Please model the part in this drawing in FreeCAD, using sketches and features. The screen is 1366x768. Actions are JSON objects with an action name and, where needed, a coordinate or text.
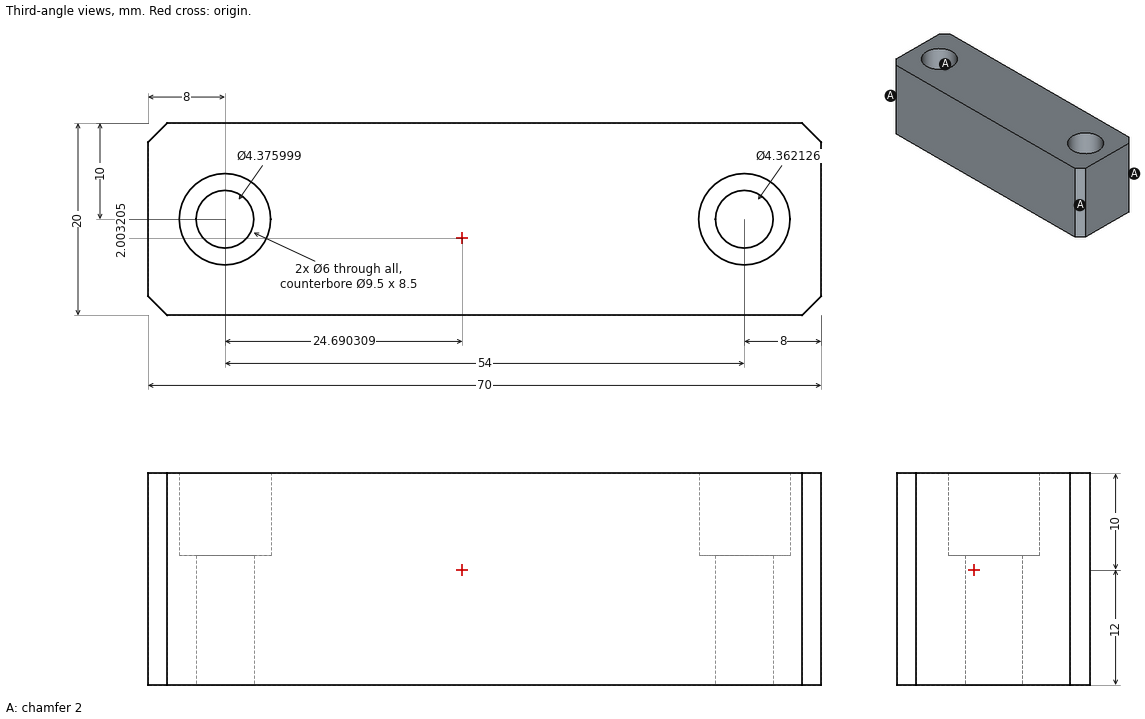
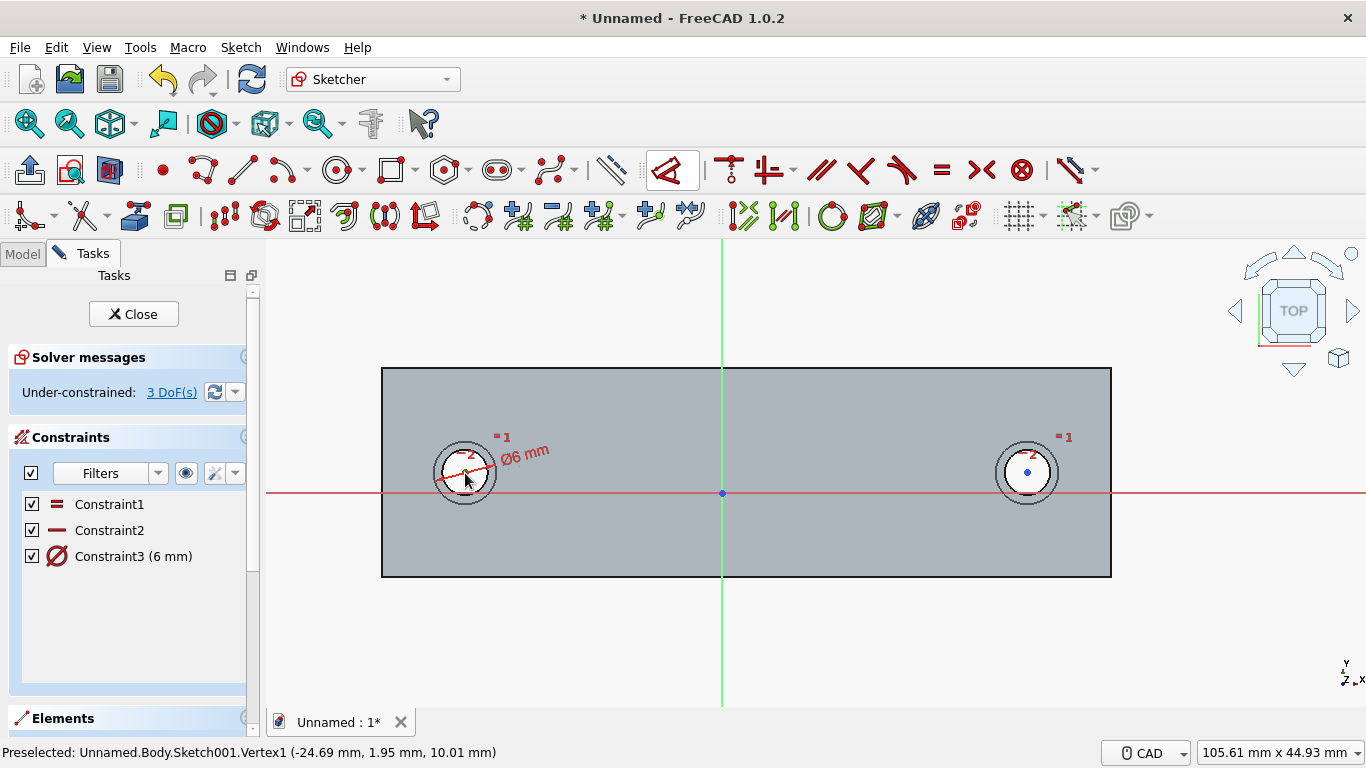
{"action": "left_click", "coordinate": [1027, 473]}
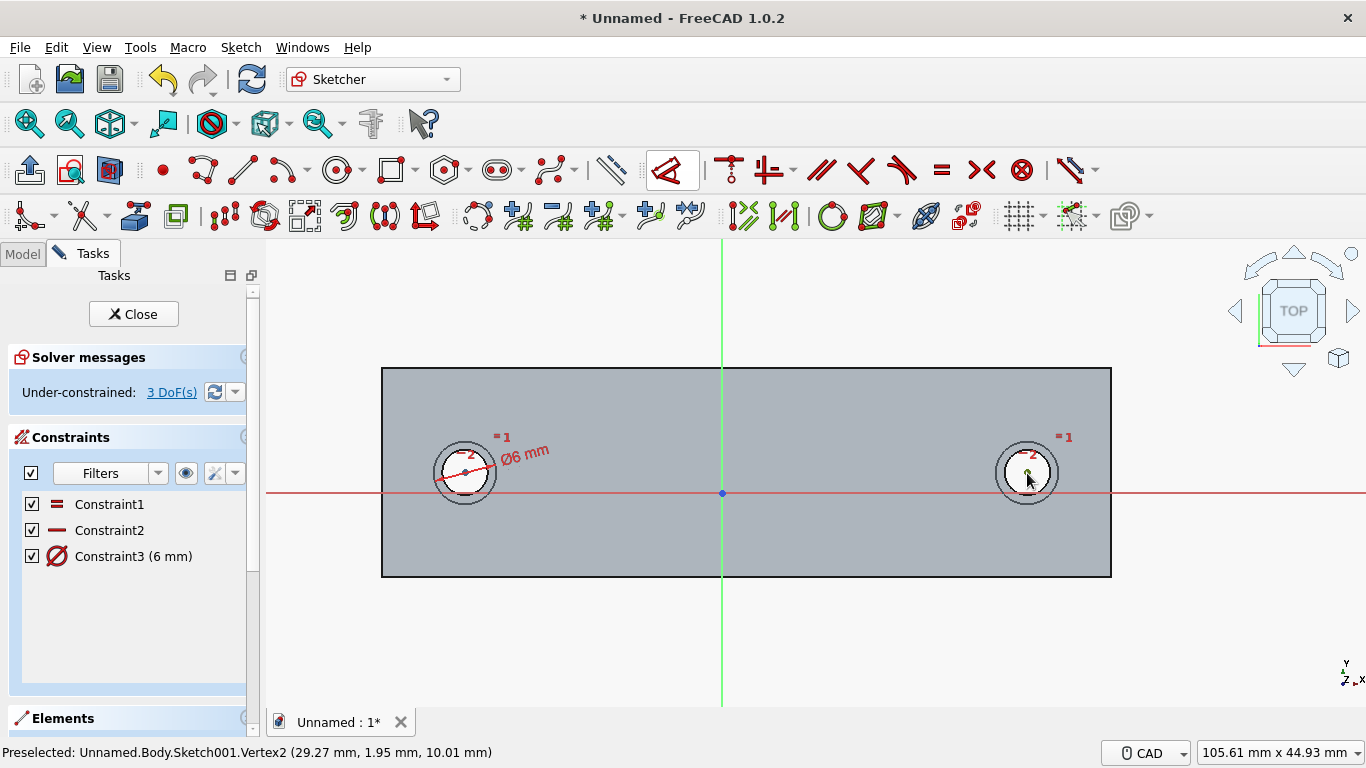
{"action": "key", "text": "l"}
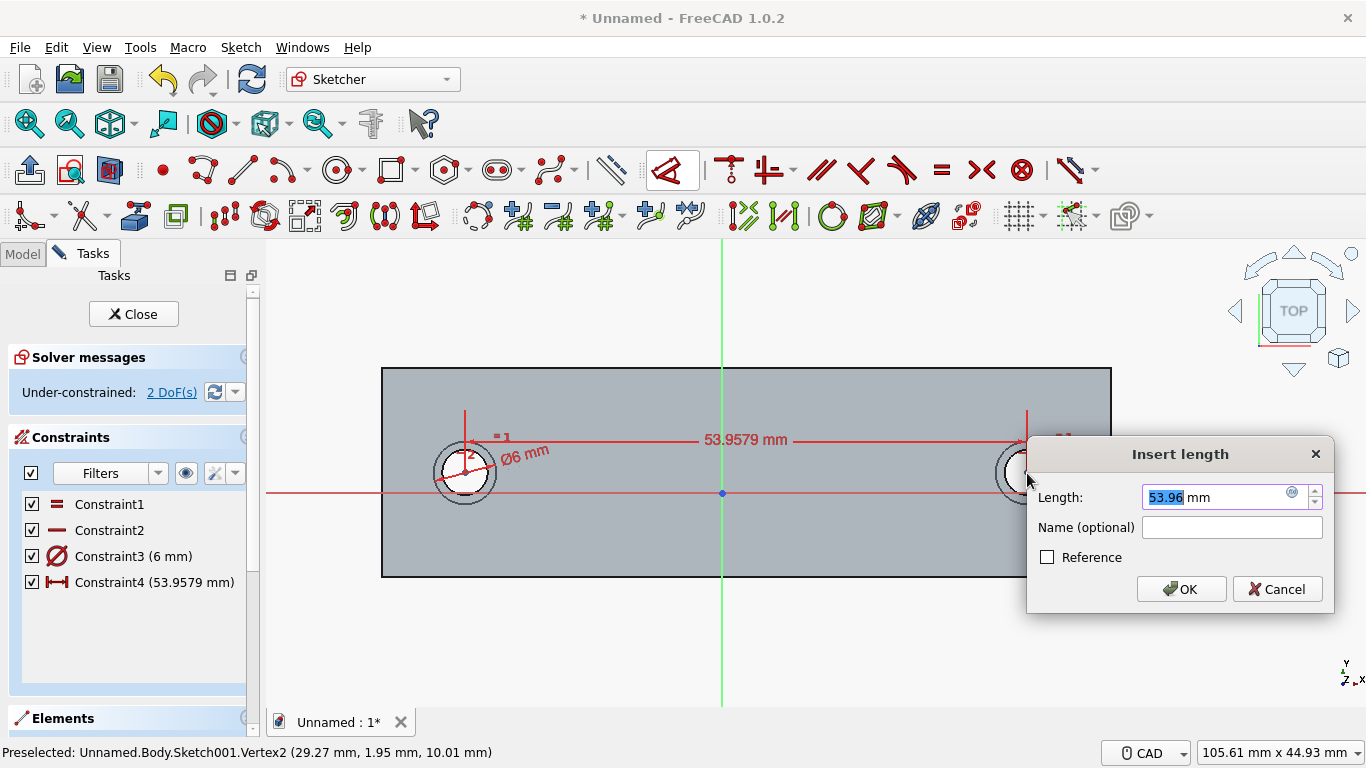
{"action": "type", "text": "54"}
{"action": "key", "text": "Return"}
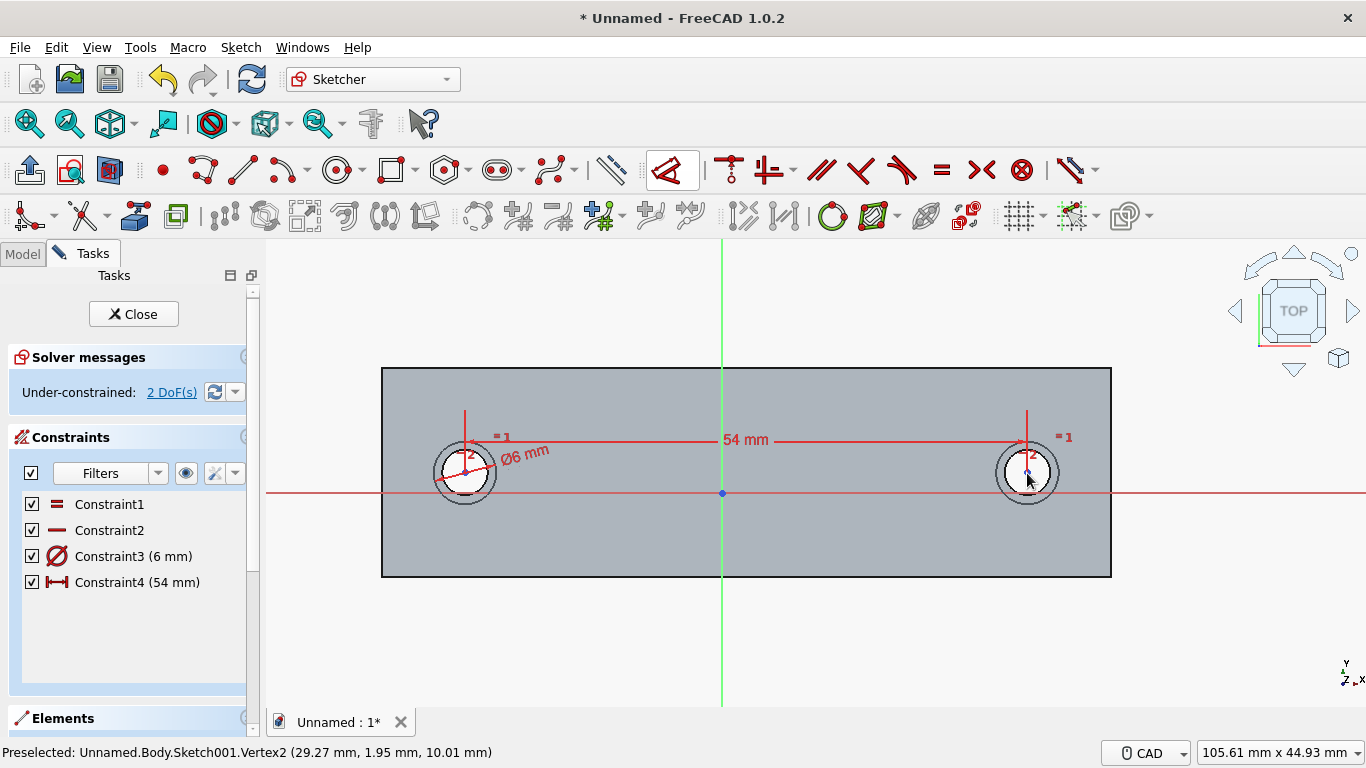
{"action": "scroll", "coordinate": [465, 473], "scroll_direction": "up", "scroll_amount": 4}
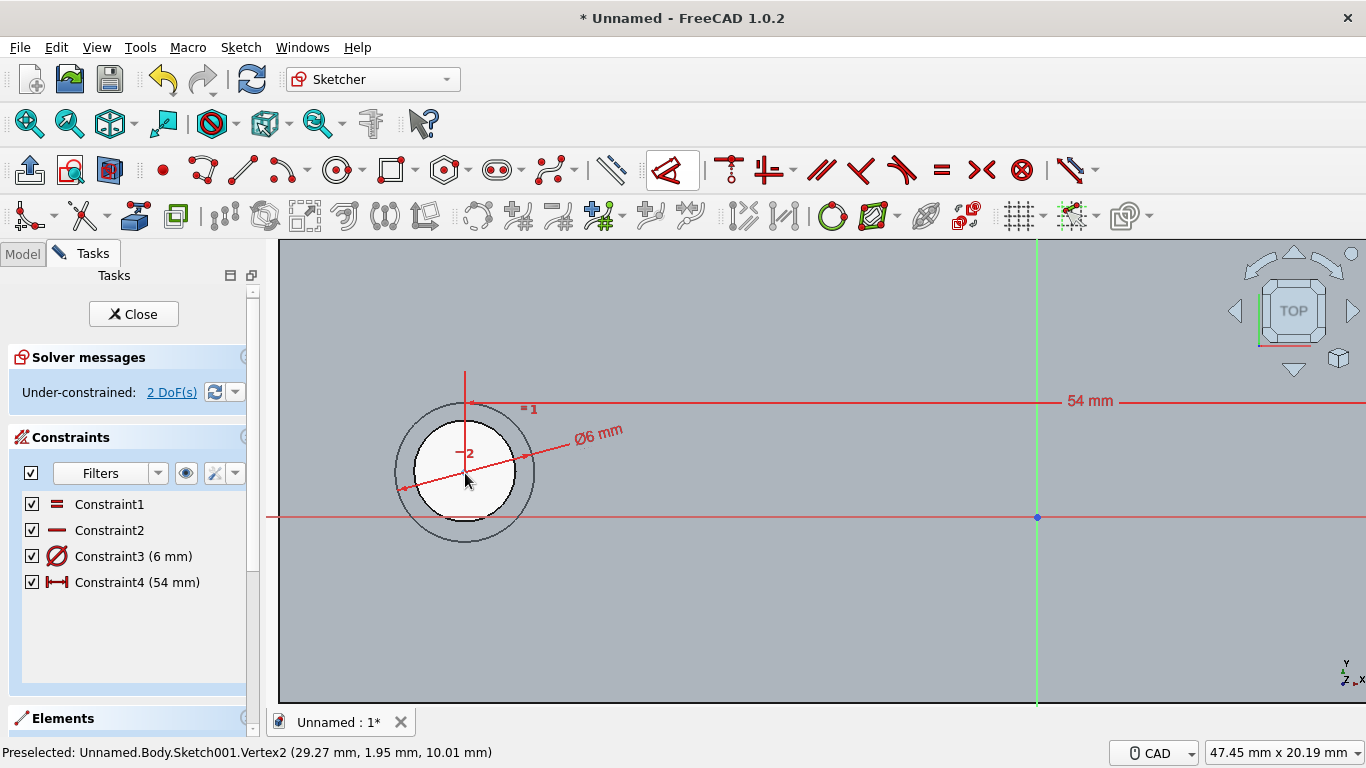
{"action": "left_click", "coordinate": [465, 472]}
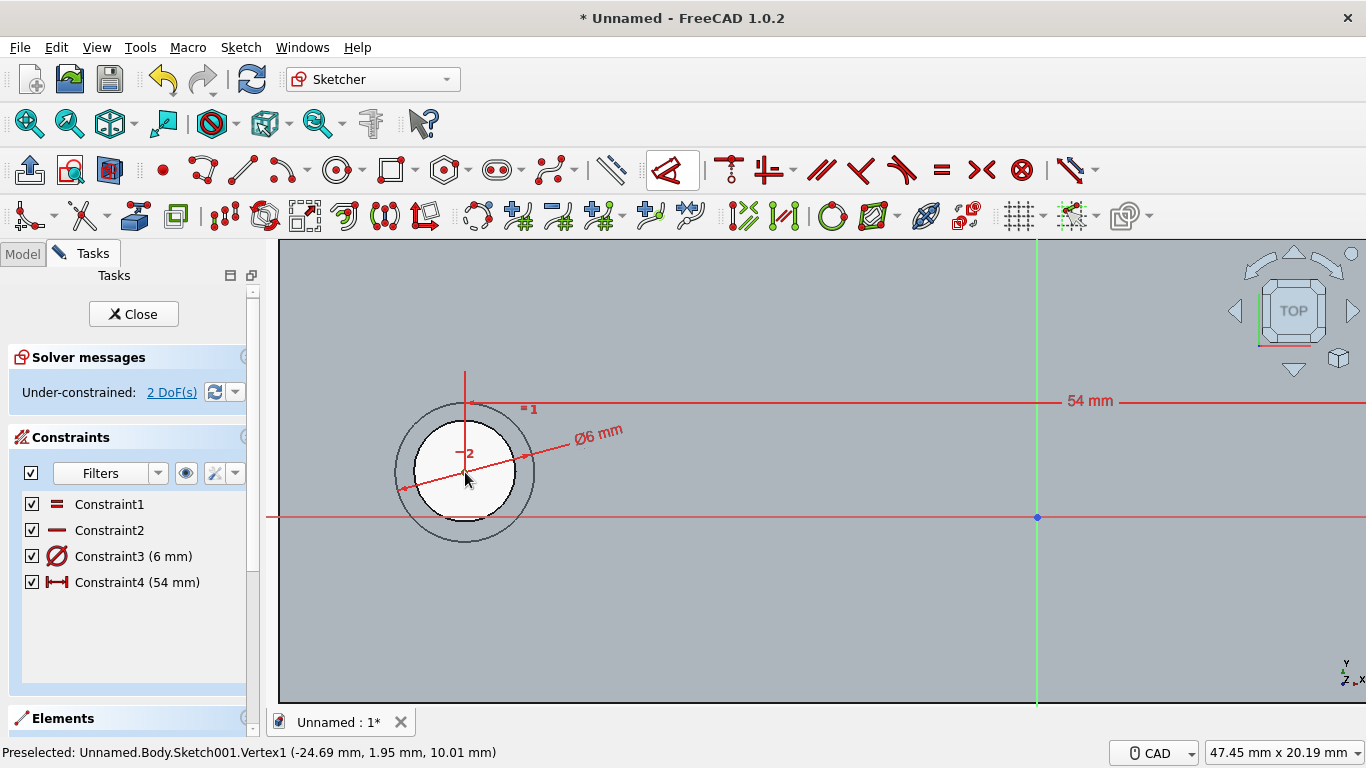
{"action": "left_click", "coordinate": [694, 170]}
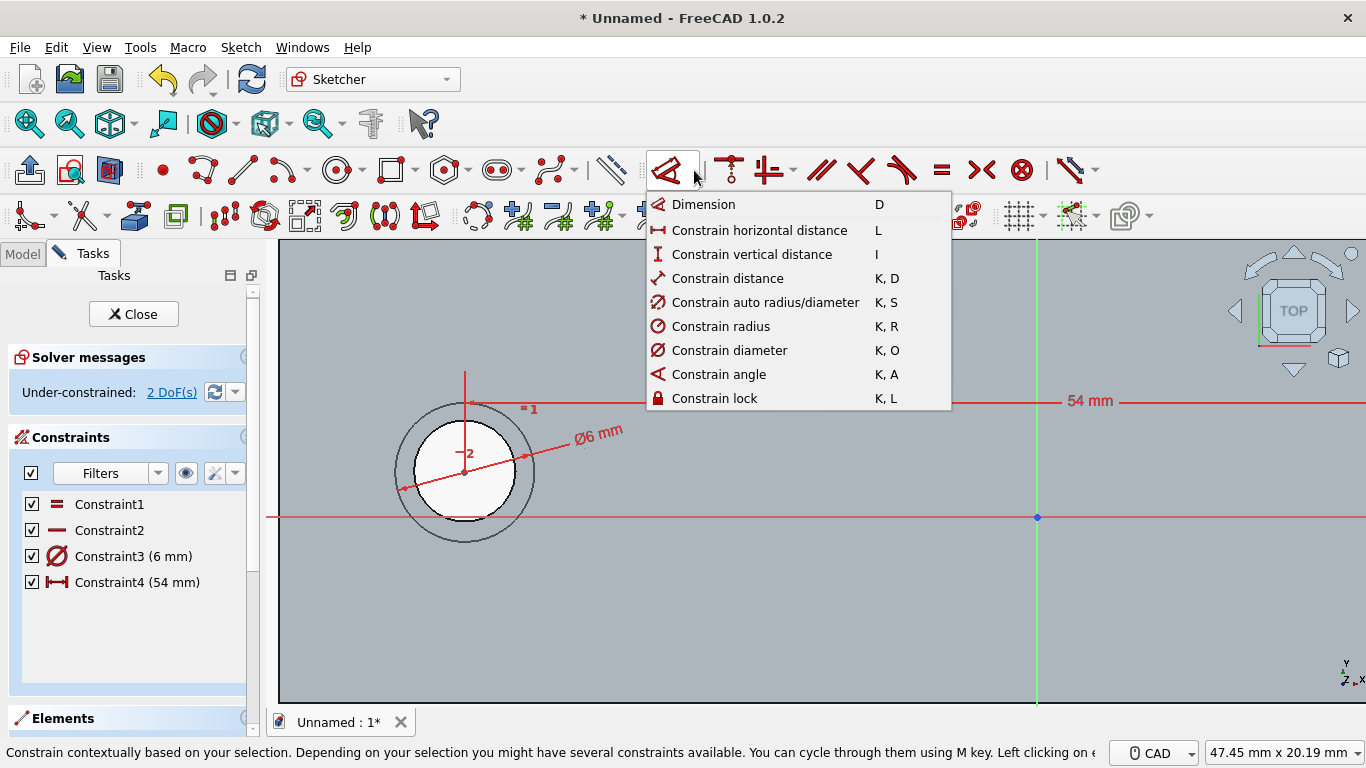
{"action": "left_click", "coordinate": [799, 254]}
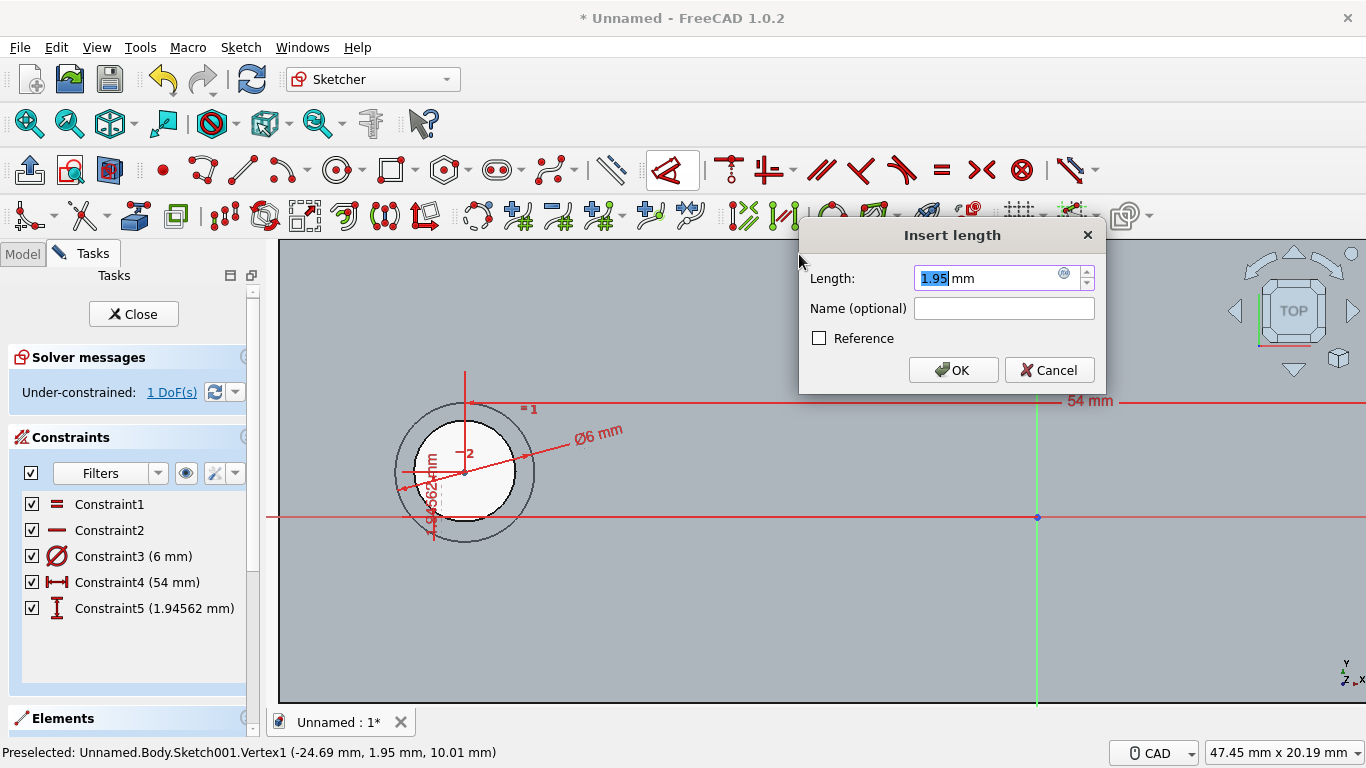
{"action": "type", "text": "2.003205"}
{"action": "key", "text": "Return"}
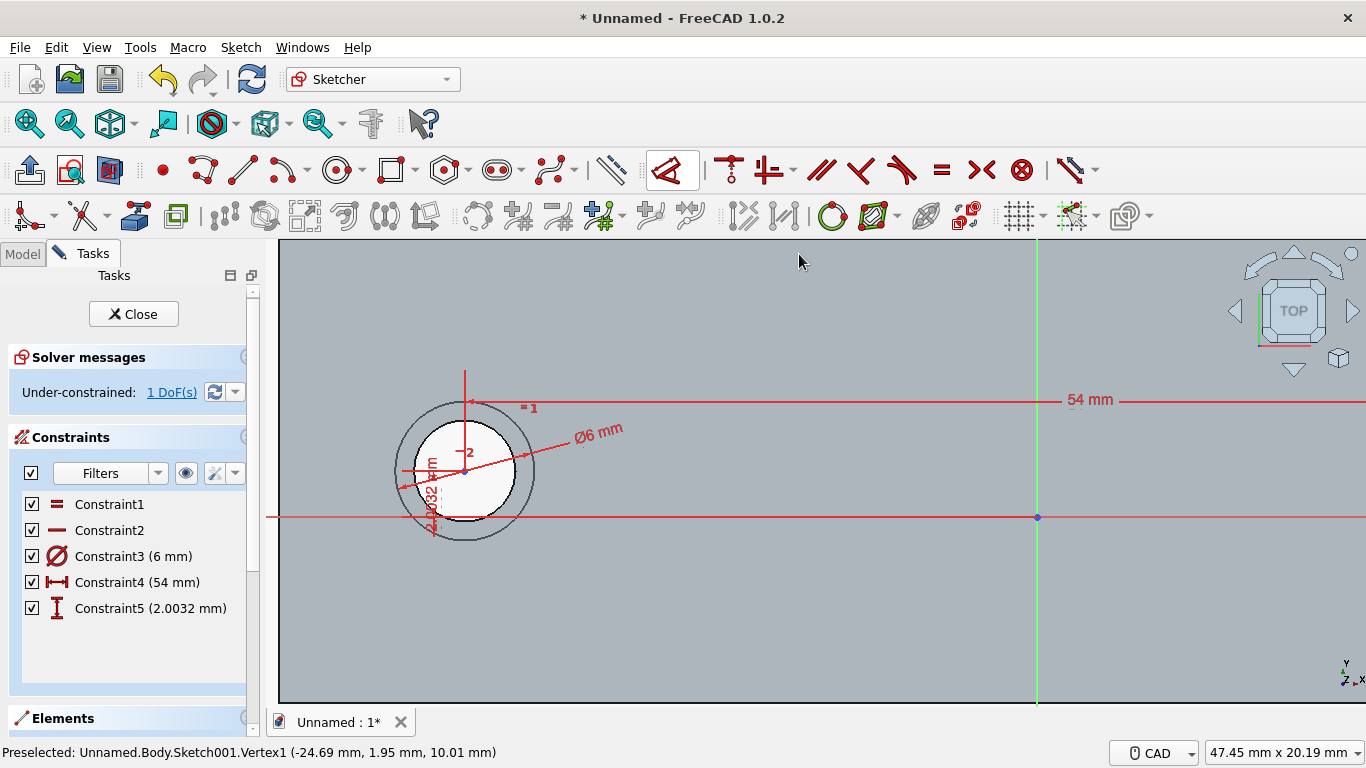
{"action": "left_click", "coordinate": [465, 471]}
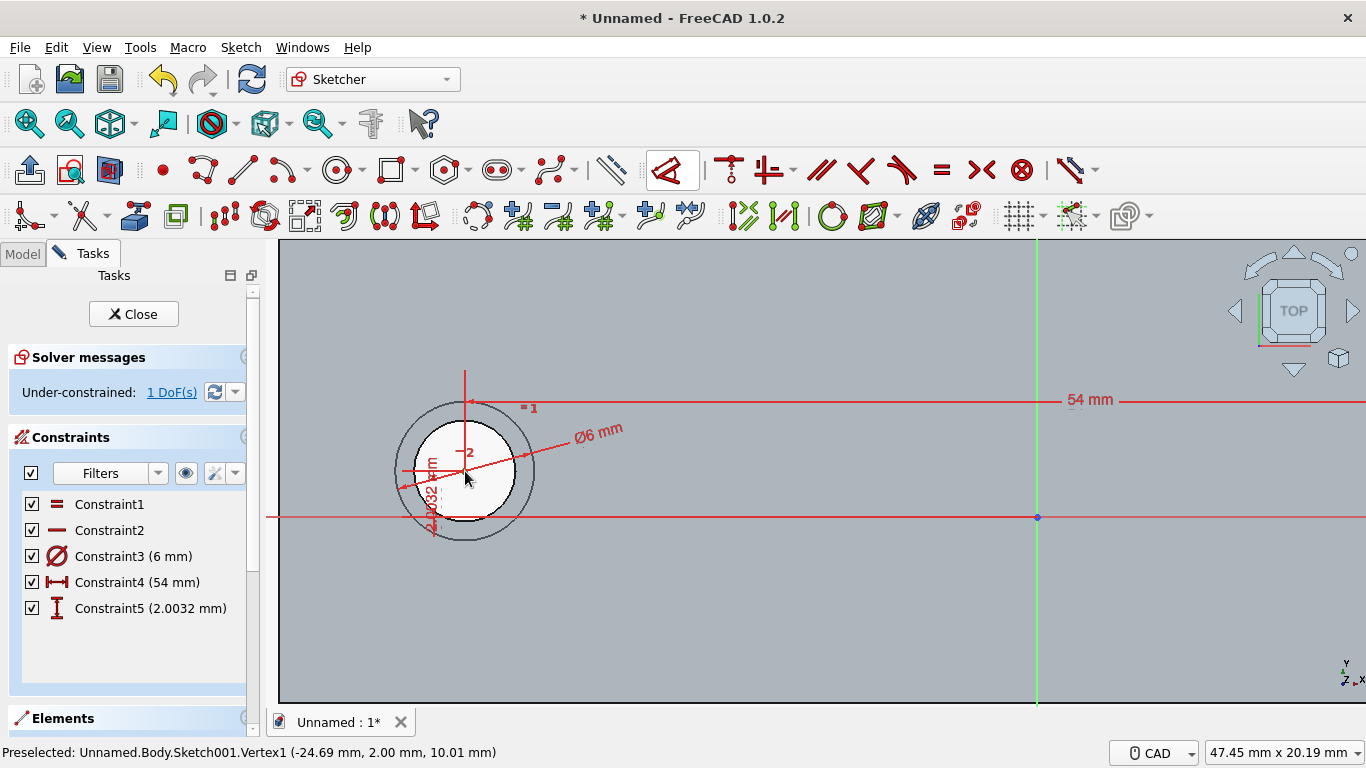
{"action": "key", "text": "l"}